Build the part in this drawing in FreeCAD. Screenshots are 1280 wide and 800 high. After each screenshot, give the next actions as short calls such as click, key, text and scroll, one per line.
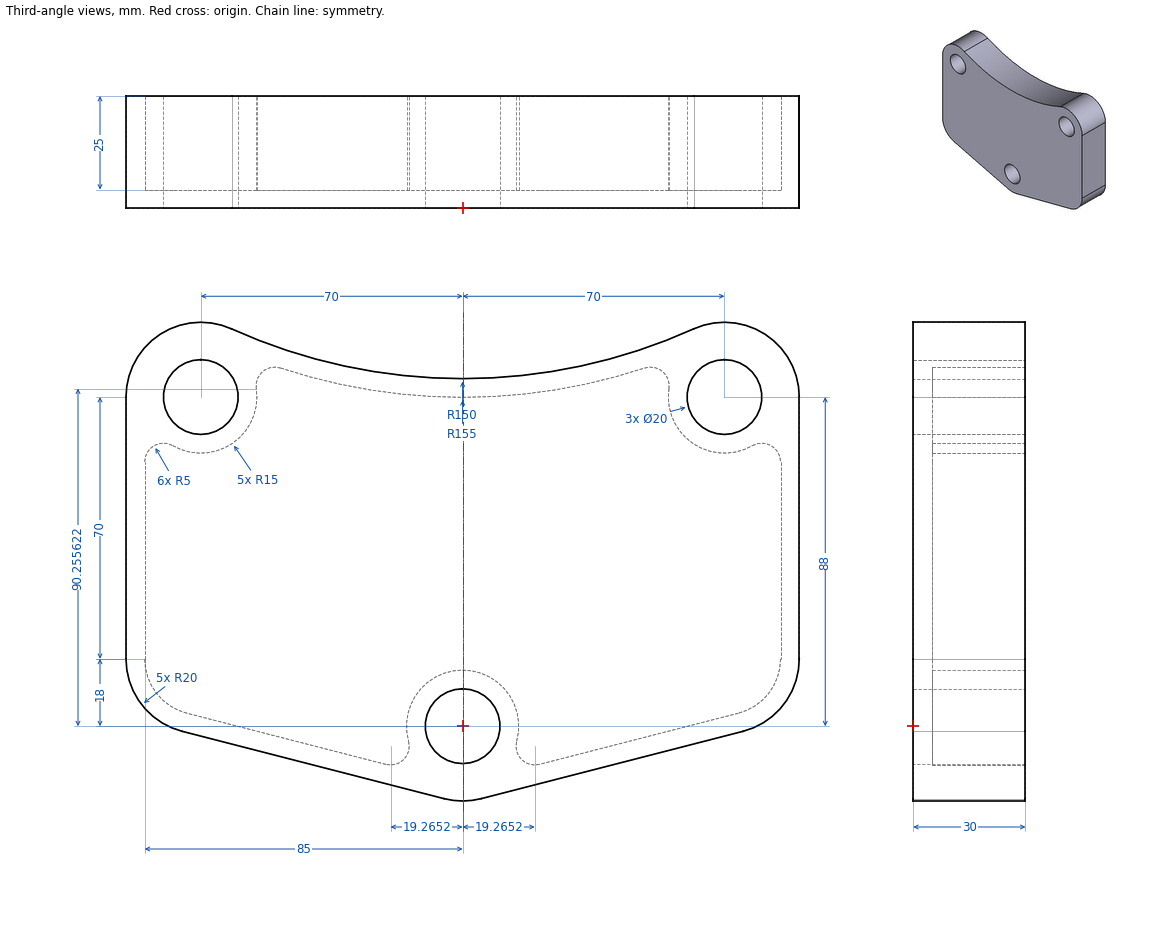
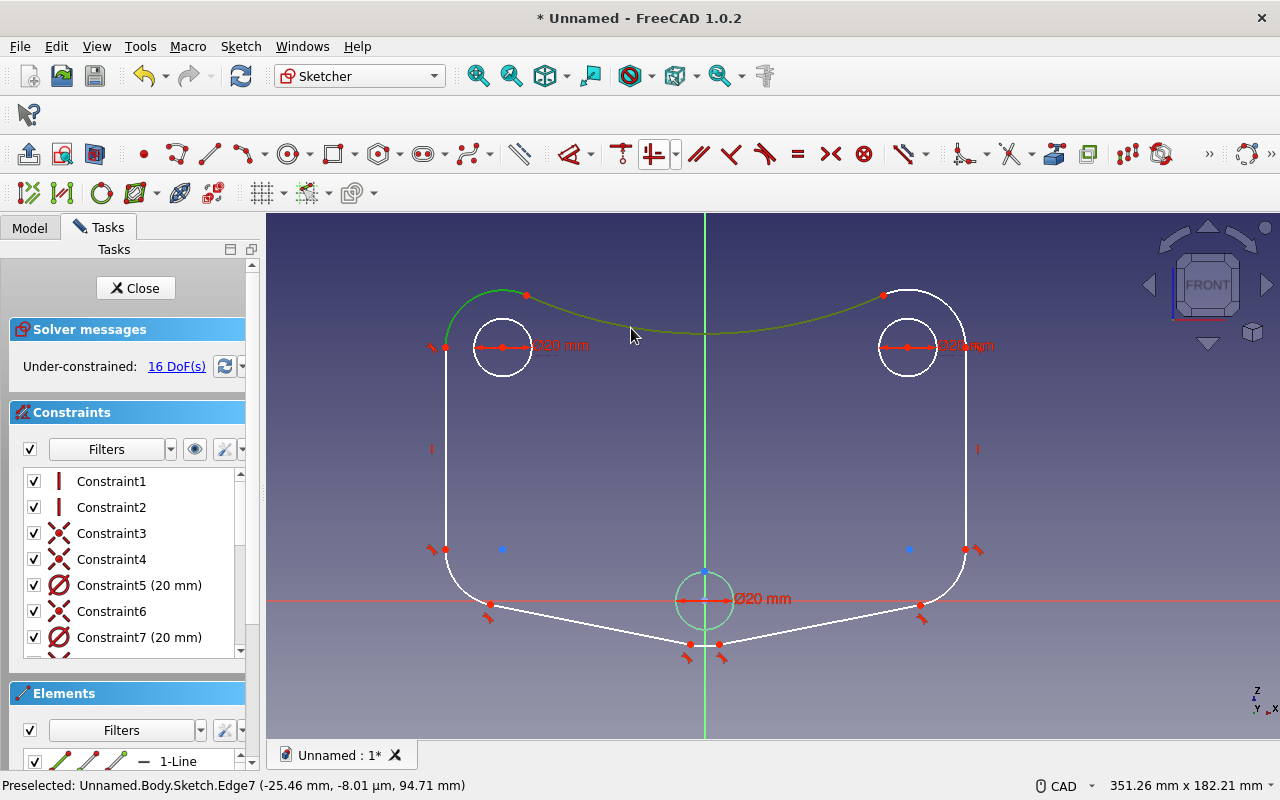
click(765, 154)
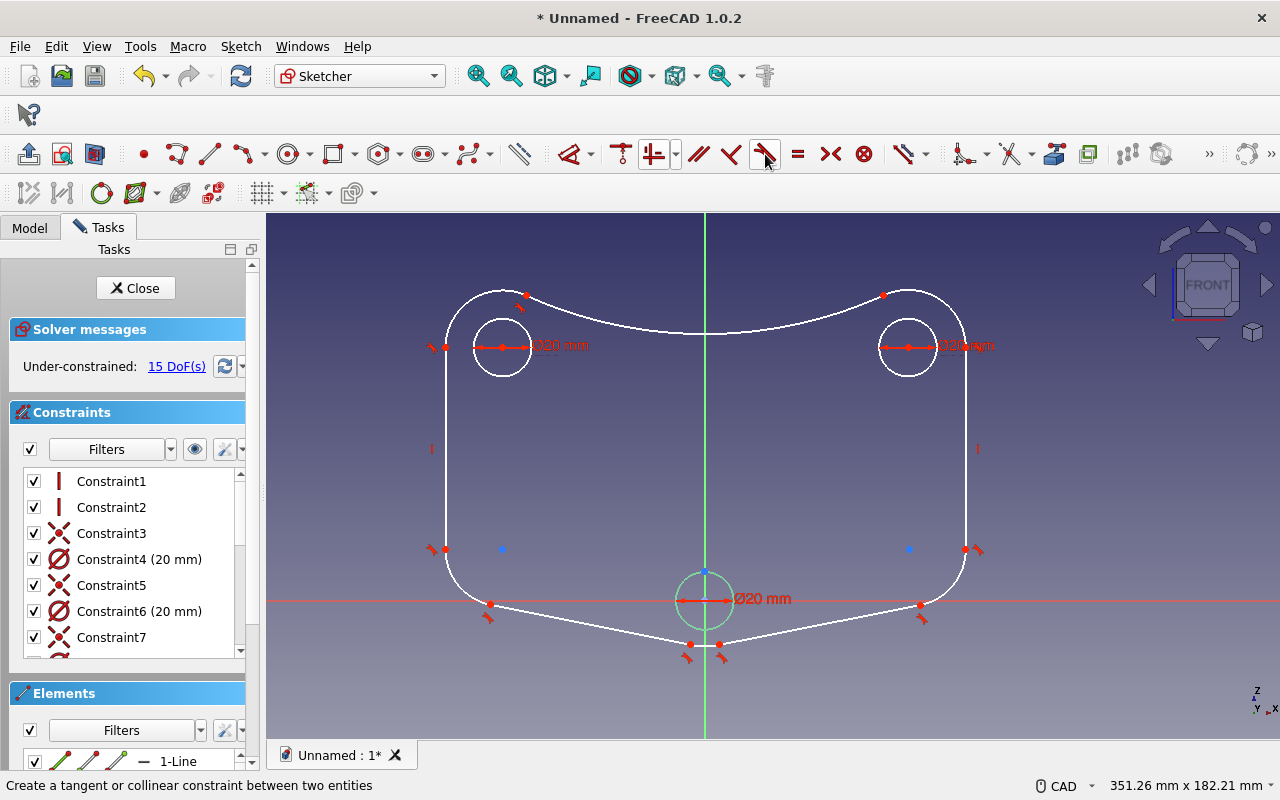
click(631, 328)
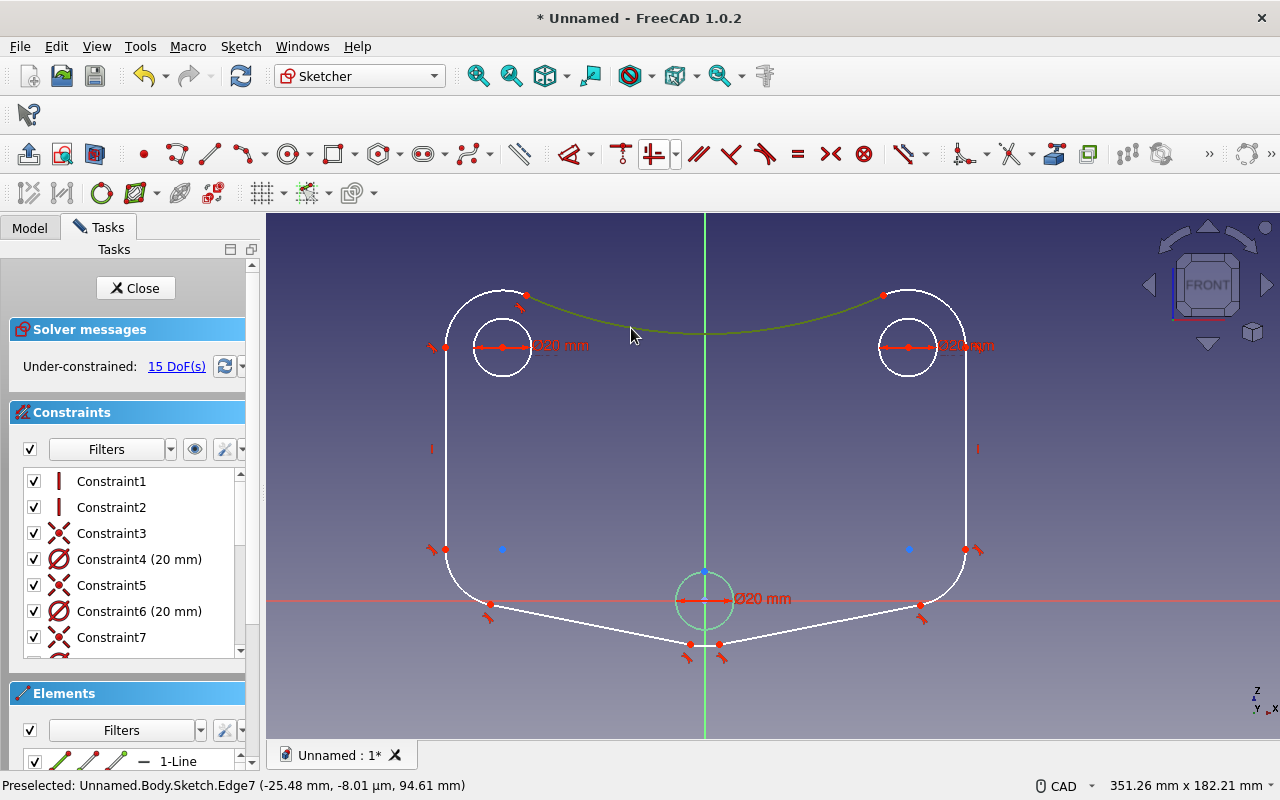
click(956, 315)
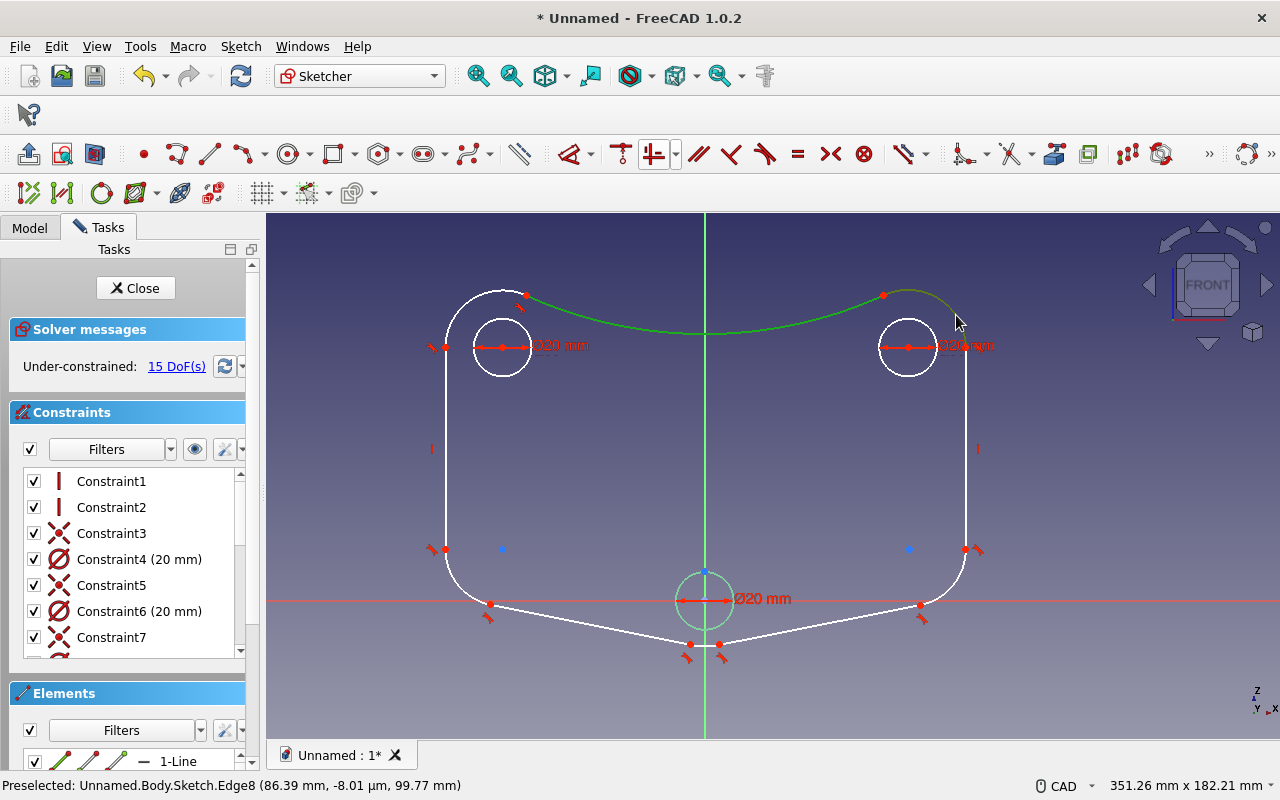
click(765, 154)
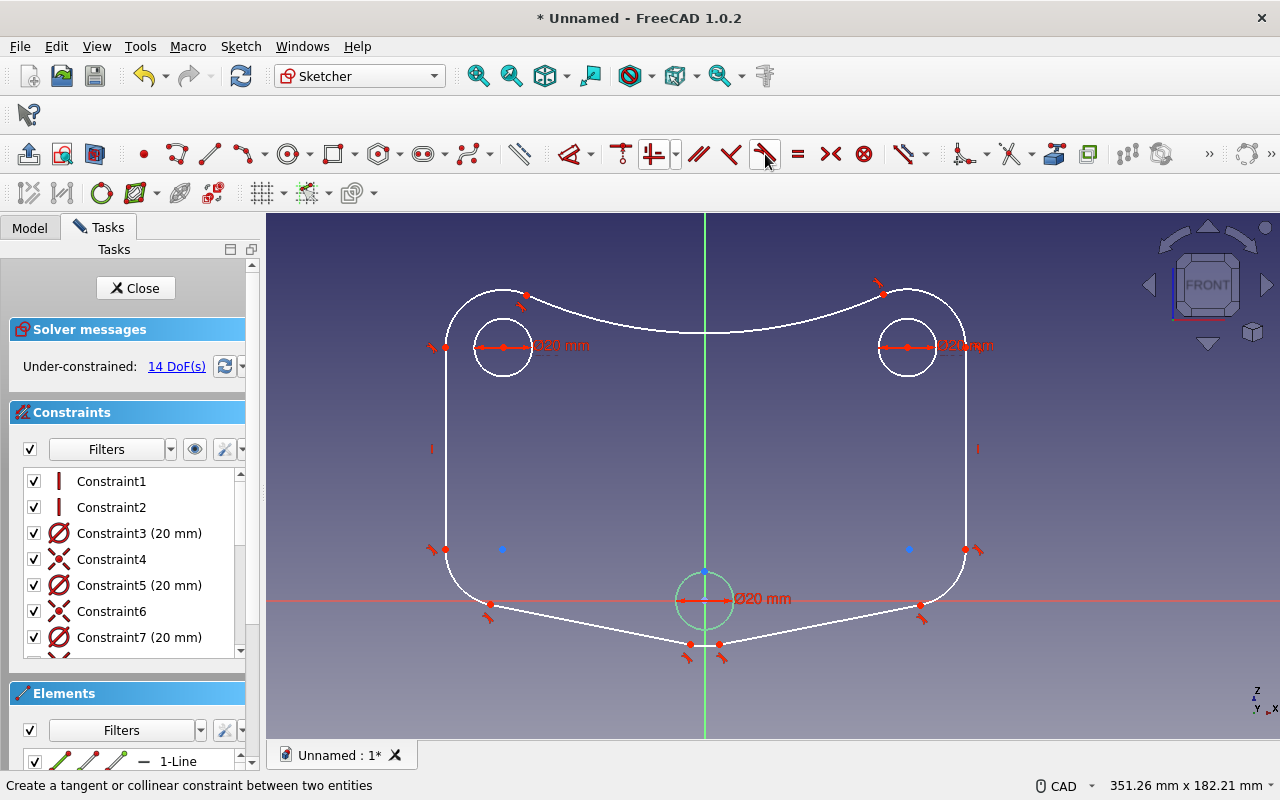
click(725, 580)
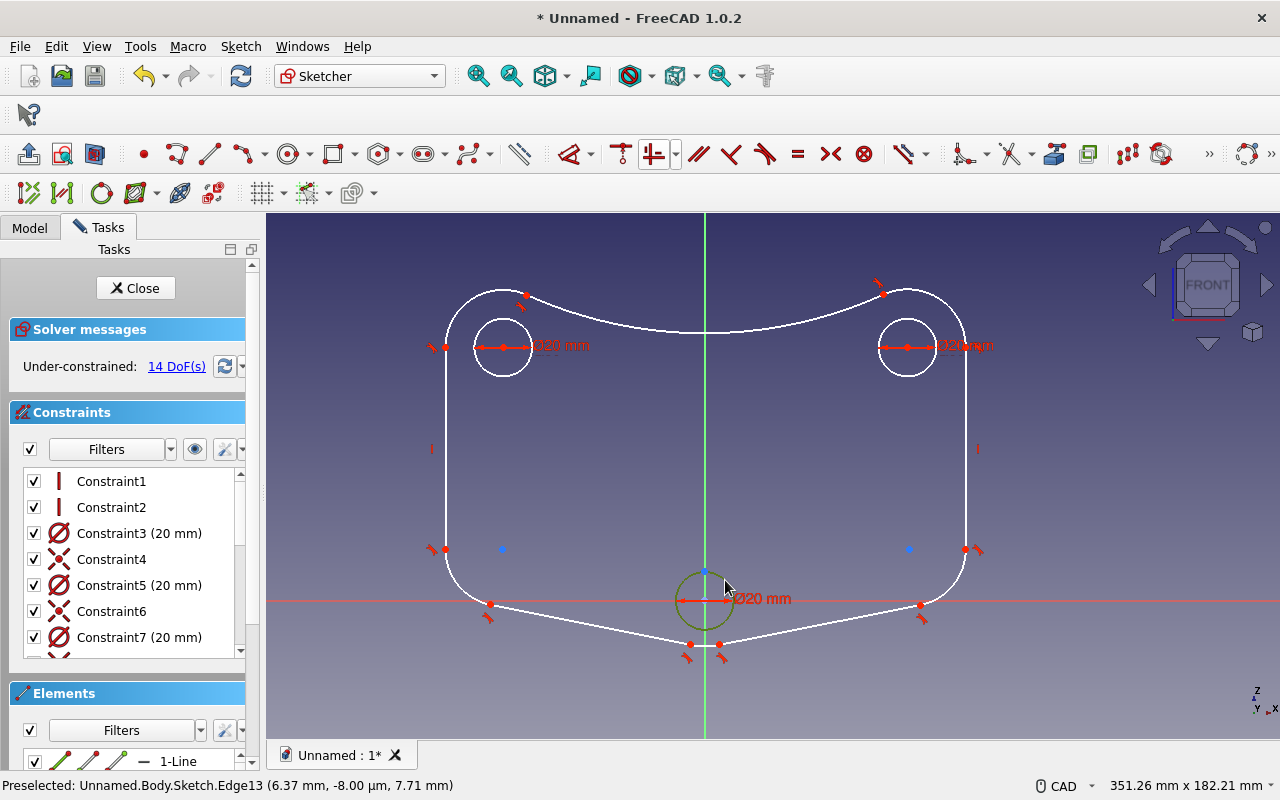
click(705, 646)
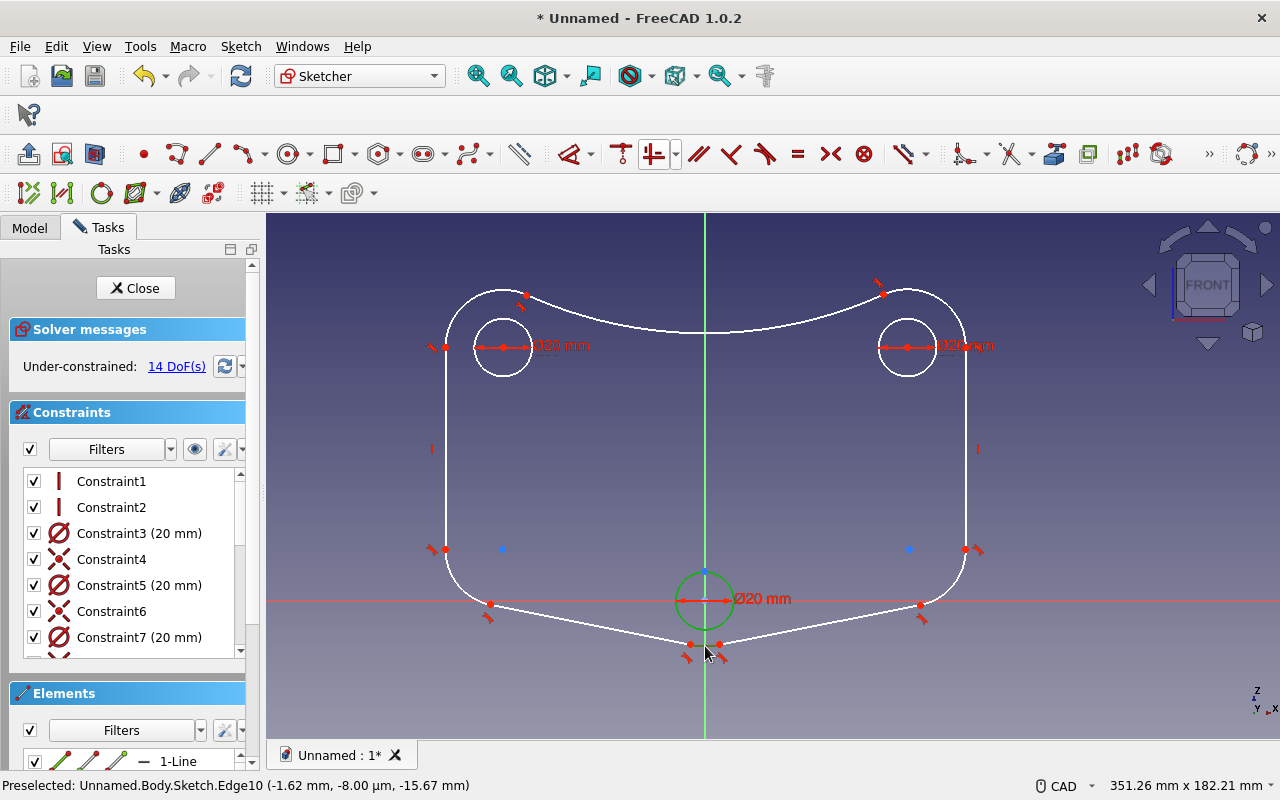
click(621, 154)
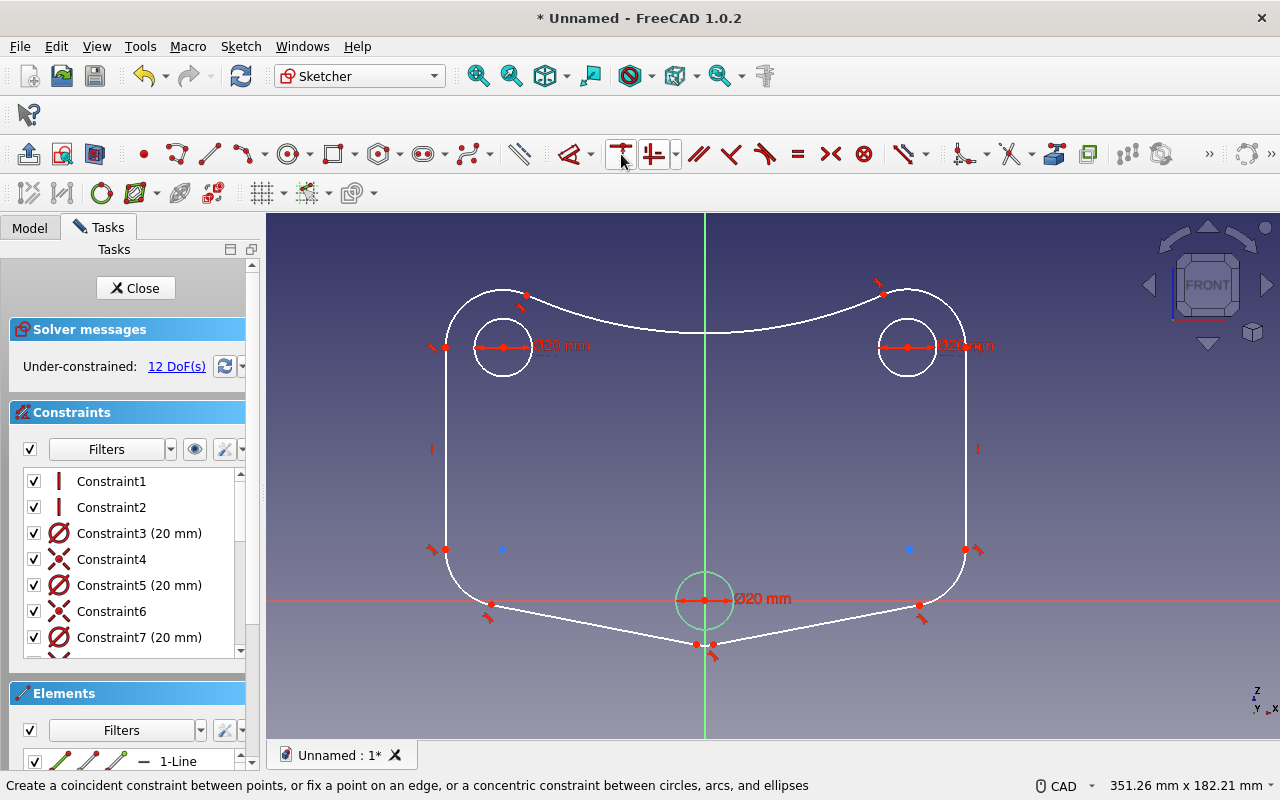
click(450, 572)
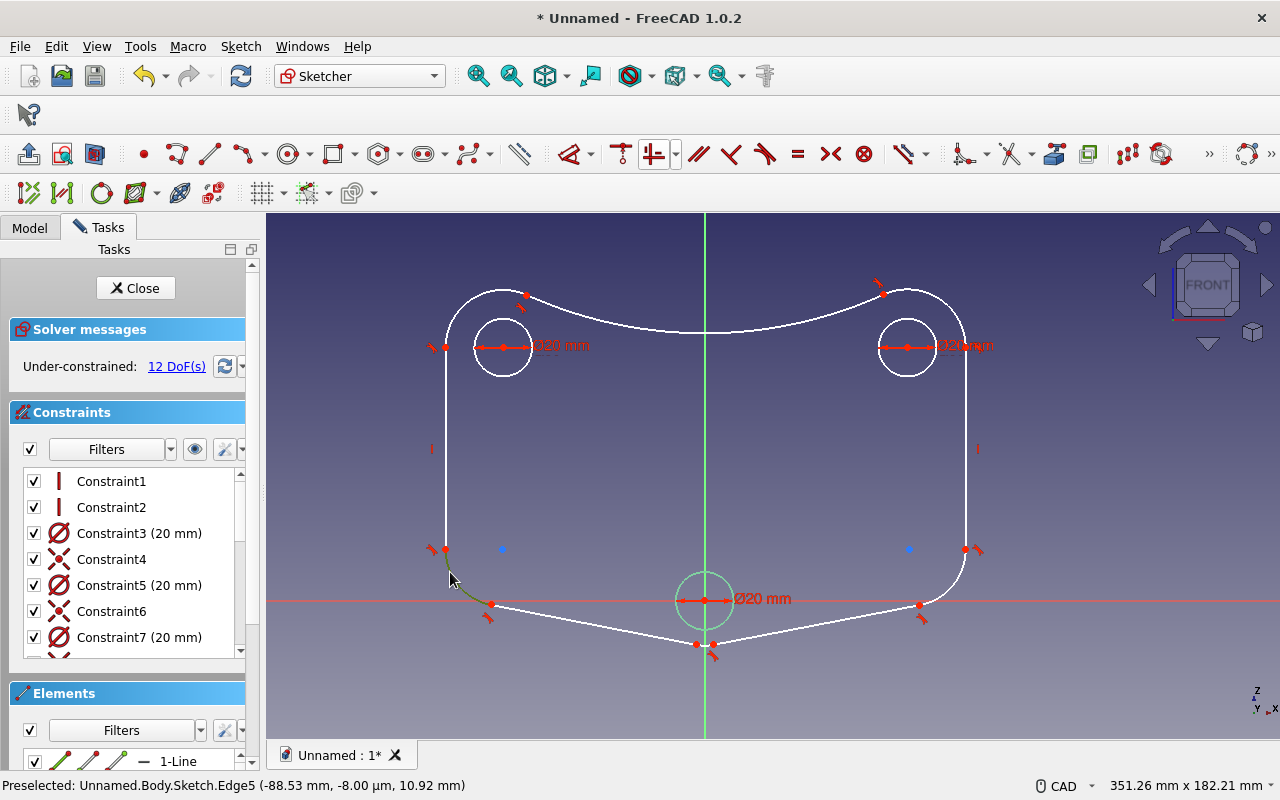
click(493, 291)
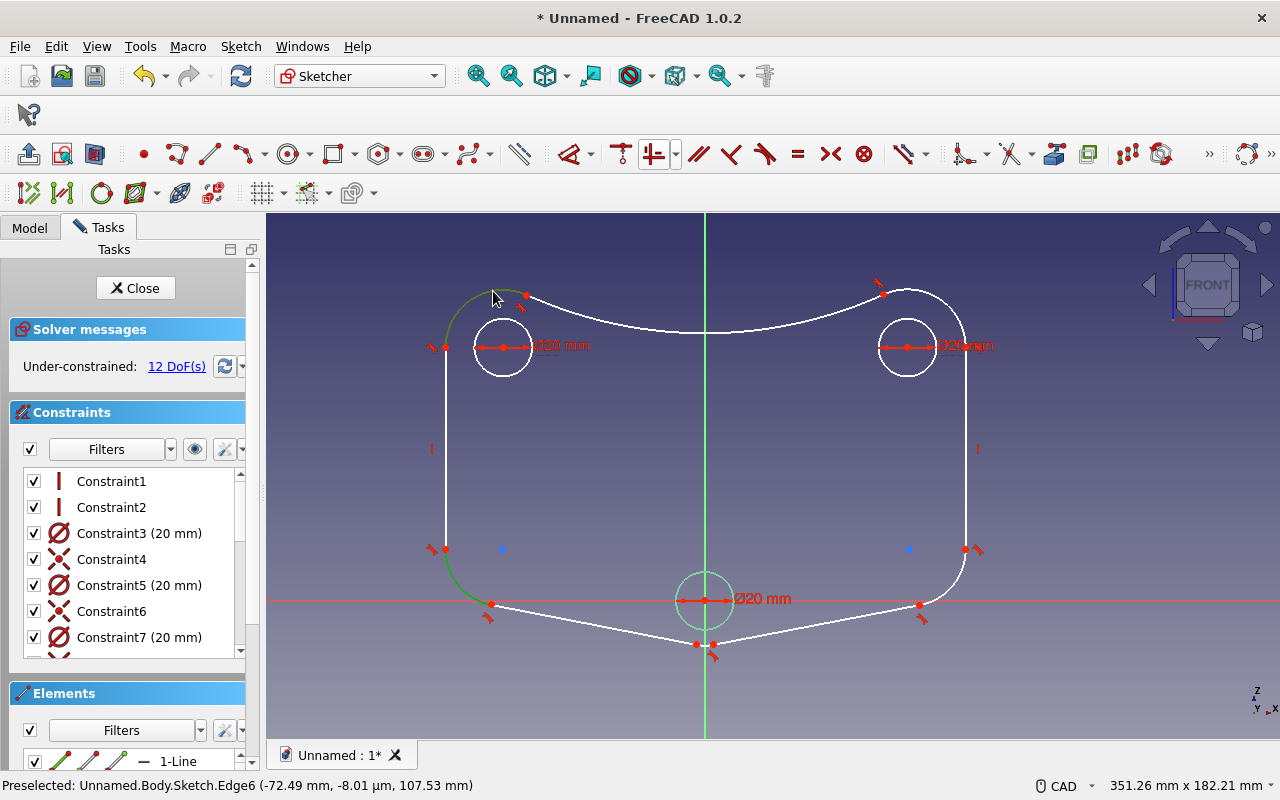
click(956, 315)